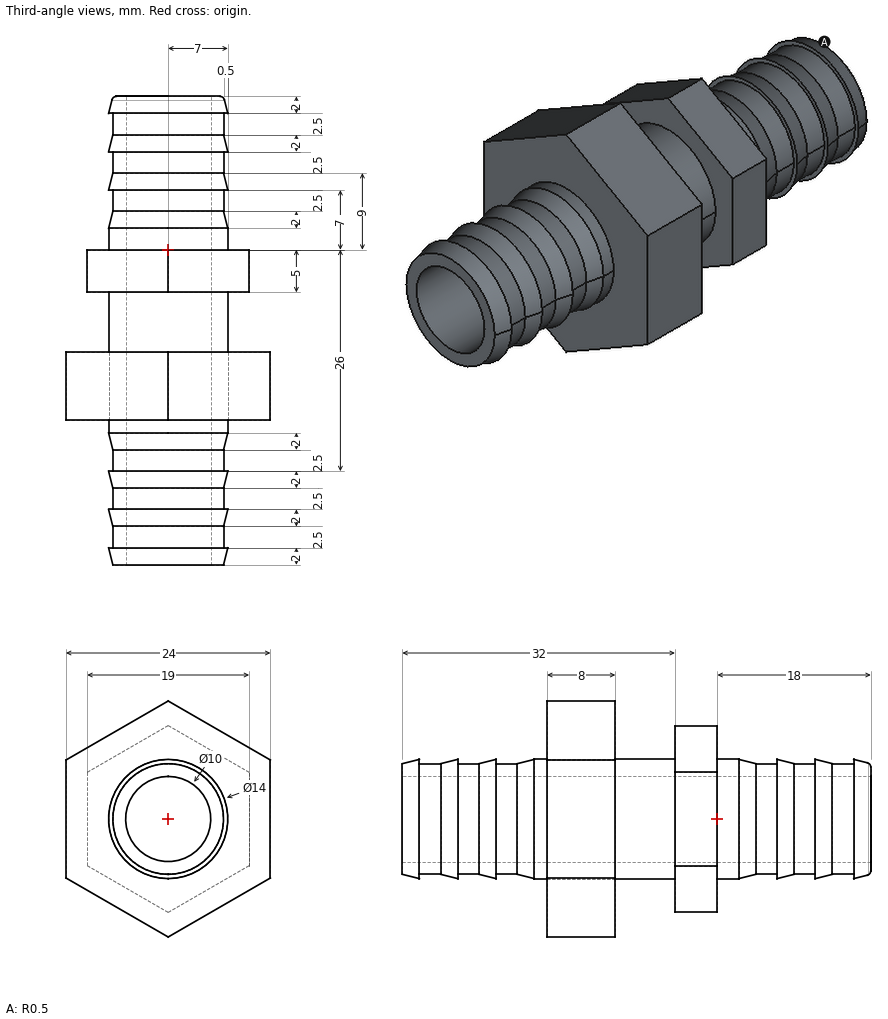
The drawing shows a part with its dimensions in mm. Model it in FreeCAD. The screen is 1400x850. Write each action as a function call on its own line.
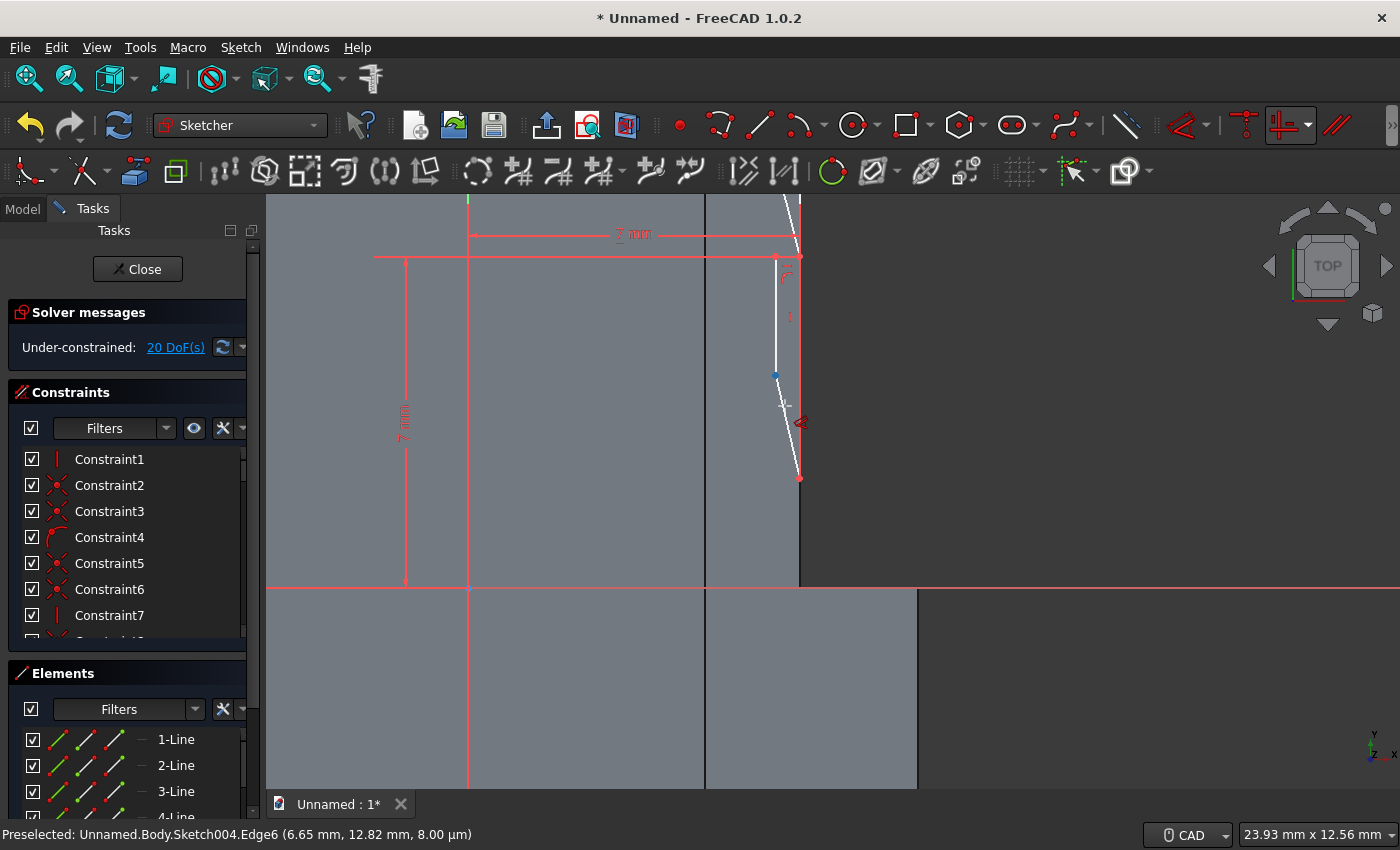
click(783, 406)
click(834, 427)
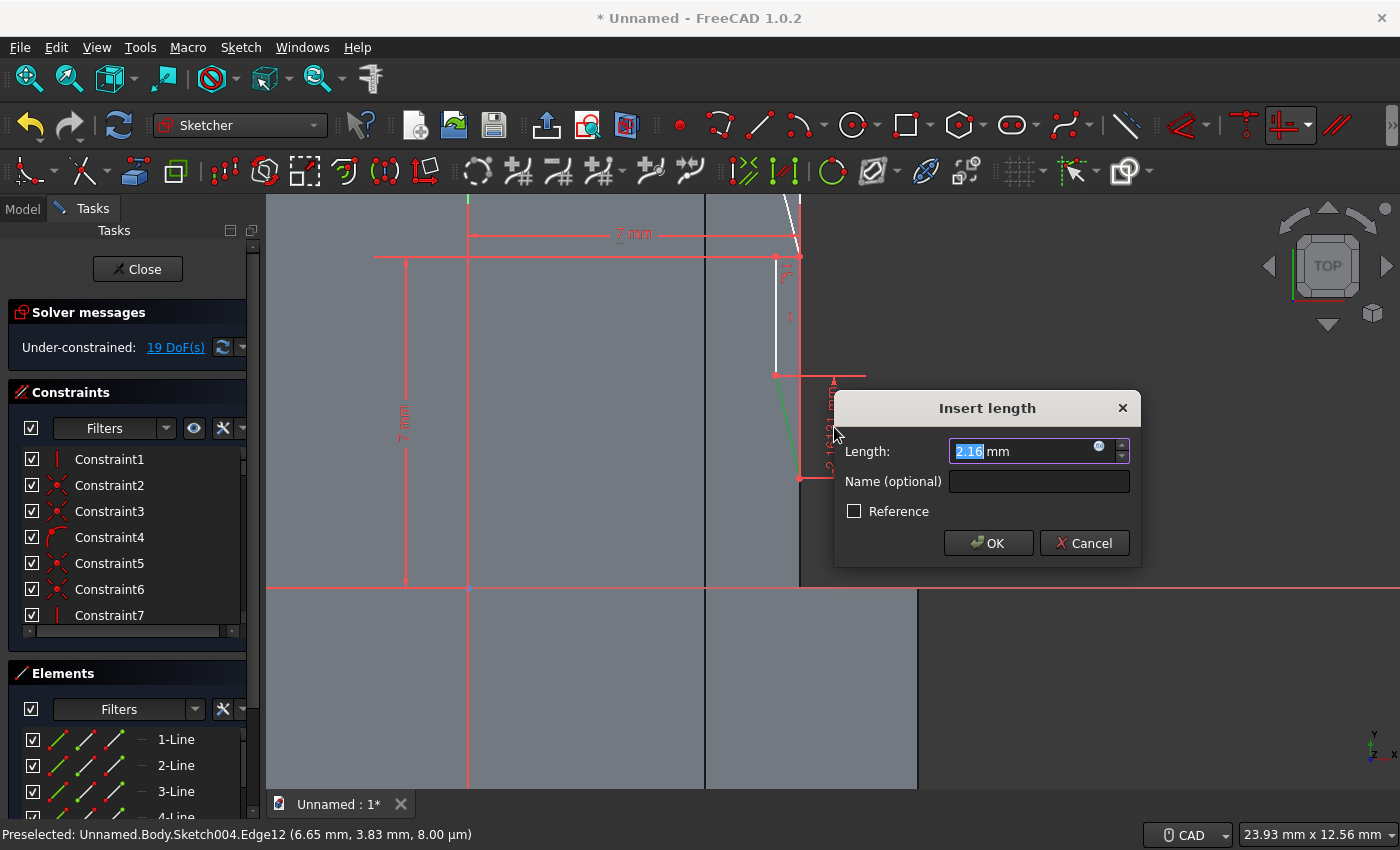
text(2)
key(Return)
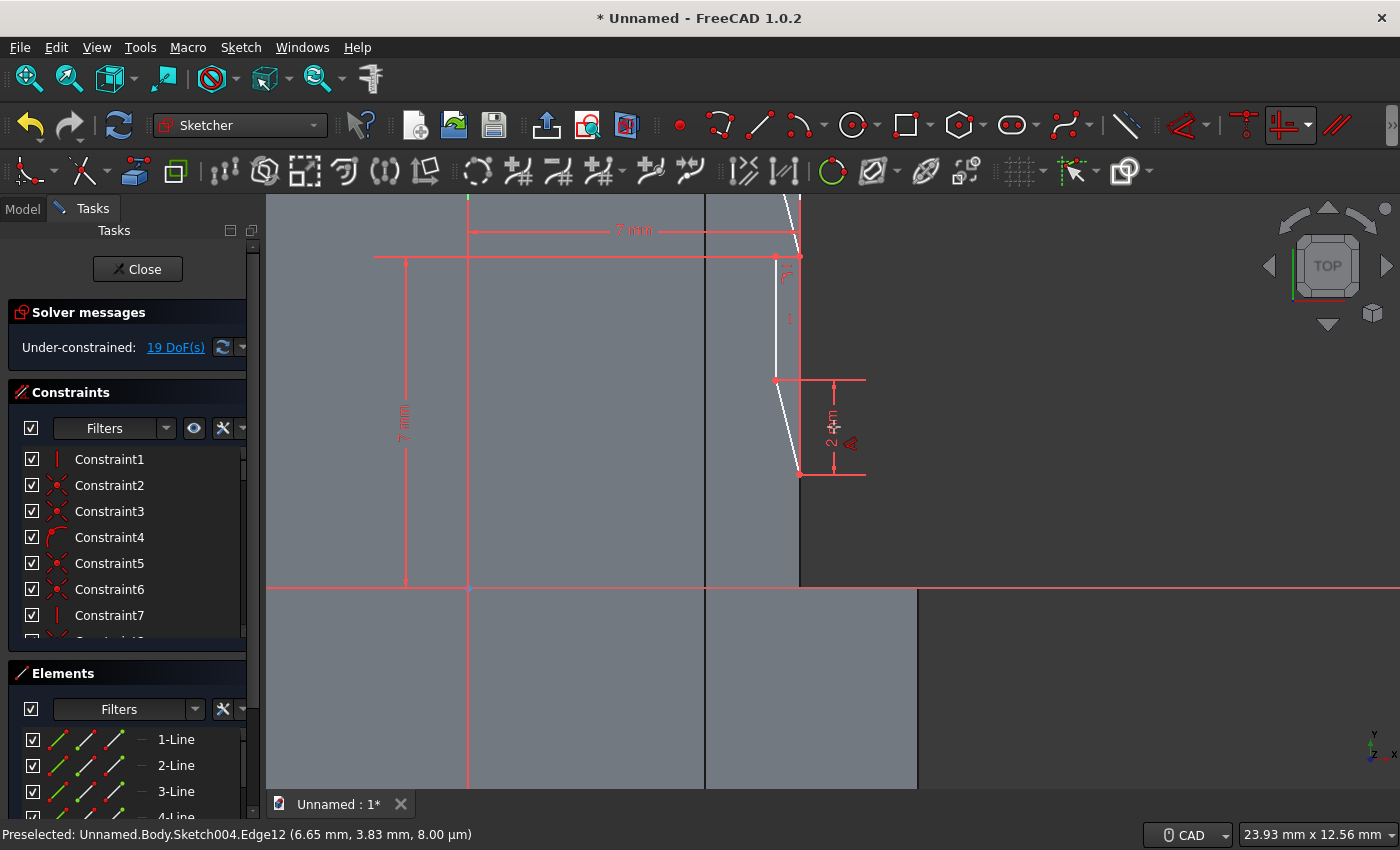
scroll(785, 406, down, 10)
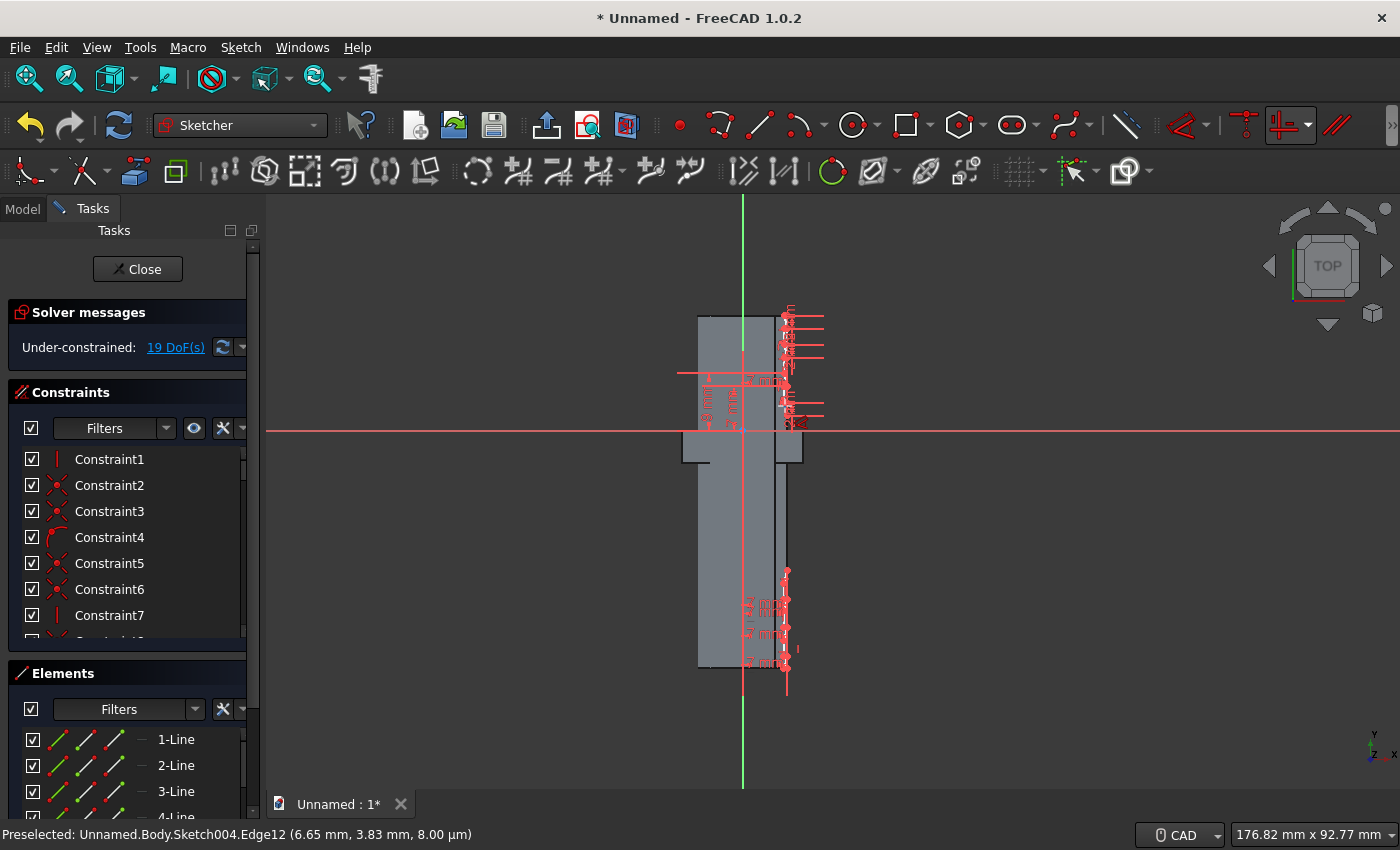
scroll(785, 579, up, 9)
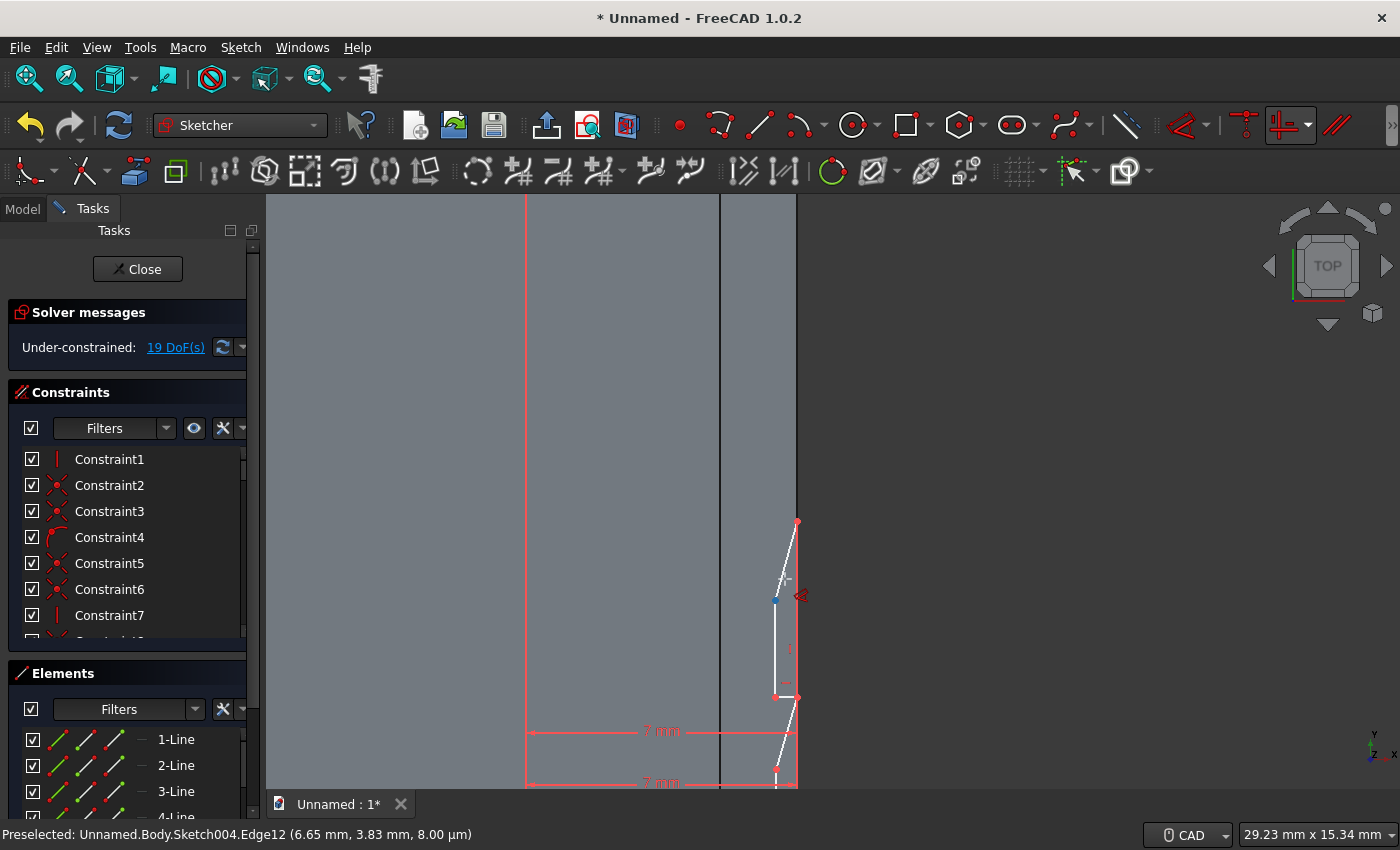
click(782, 577)
click(831, 561)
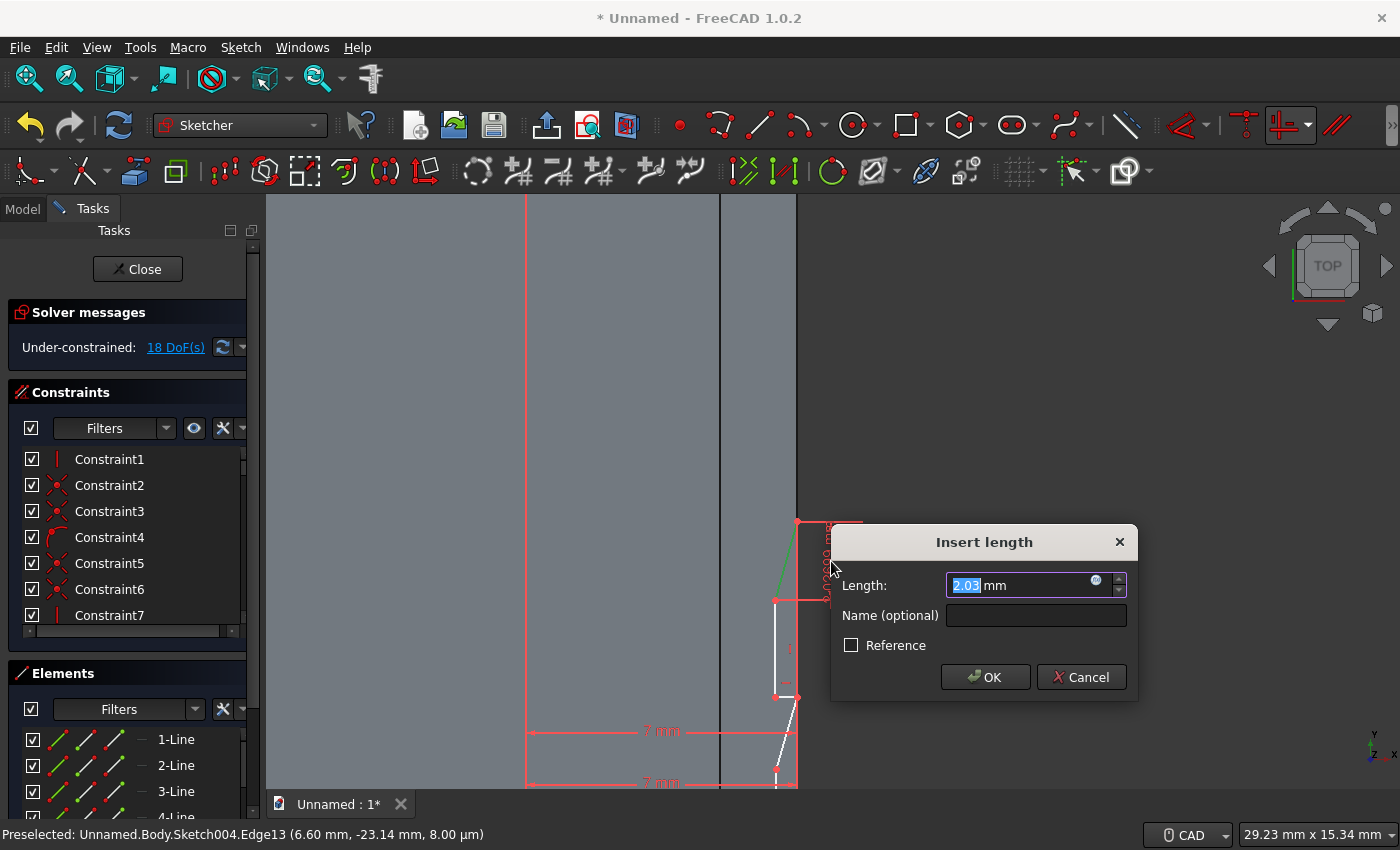
text(2)
key(Return)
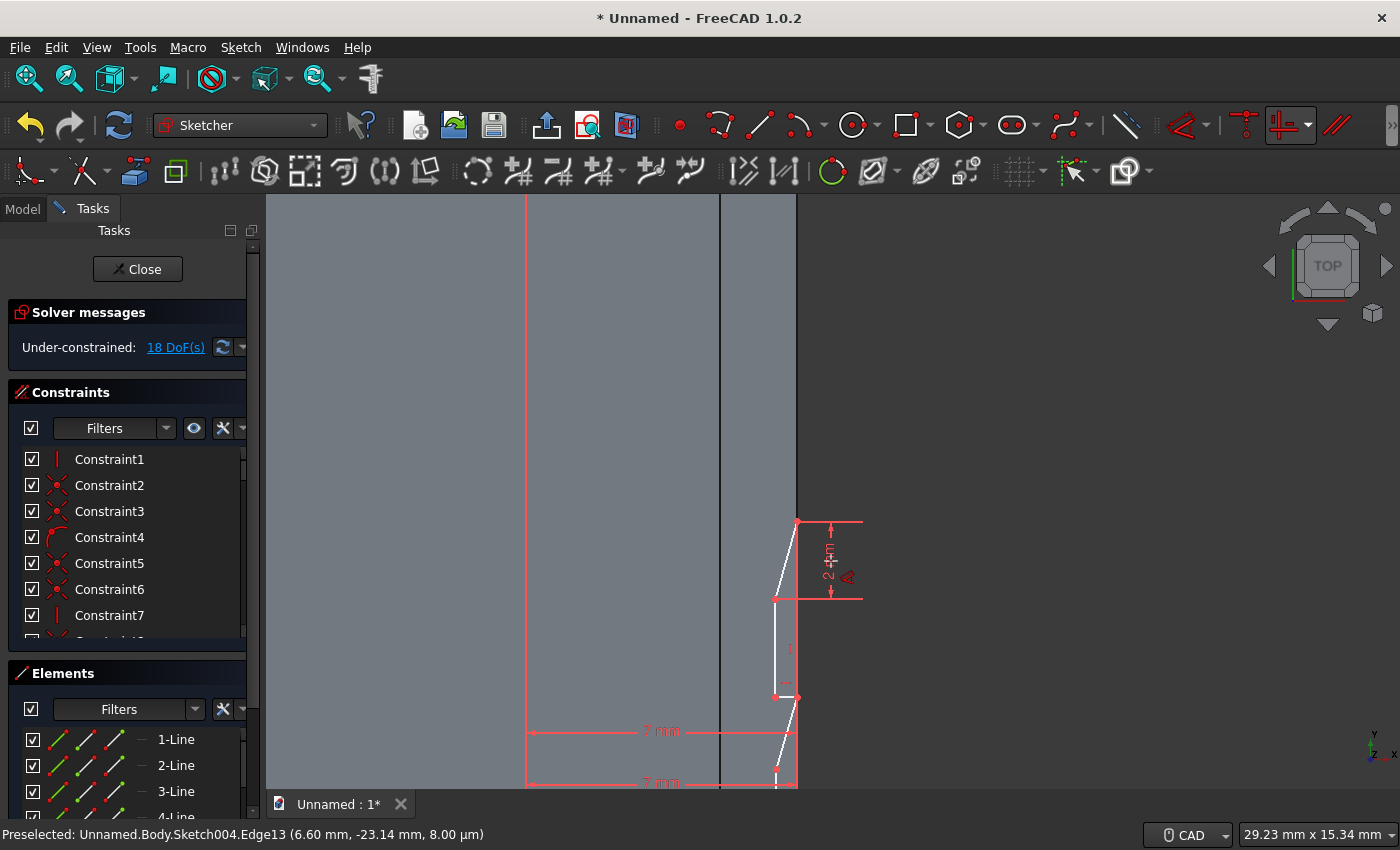
click(783, 748)
click(831, 729)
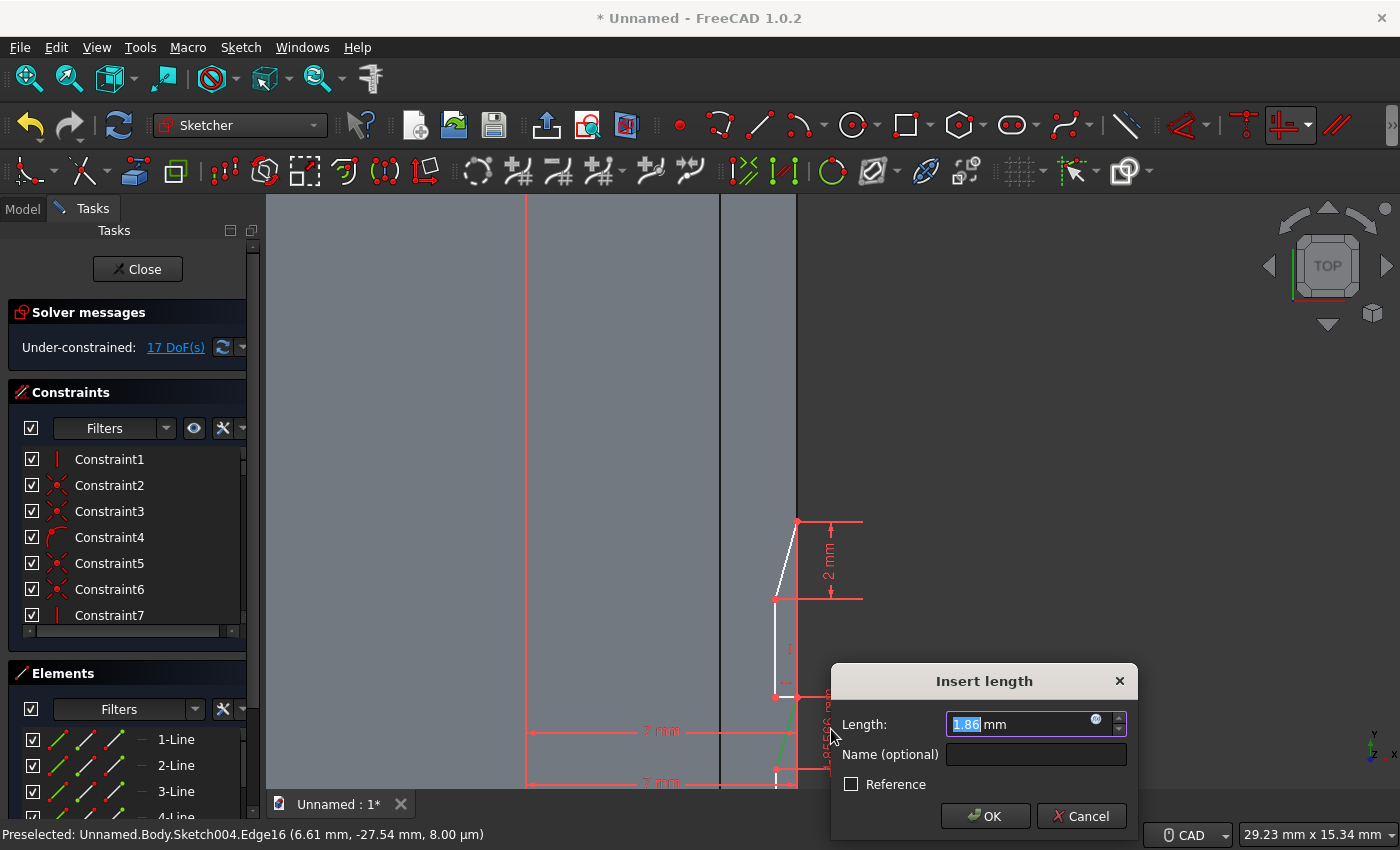
text(2)
key(Return)